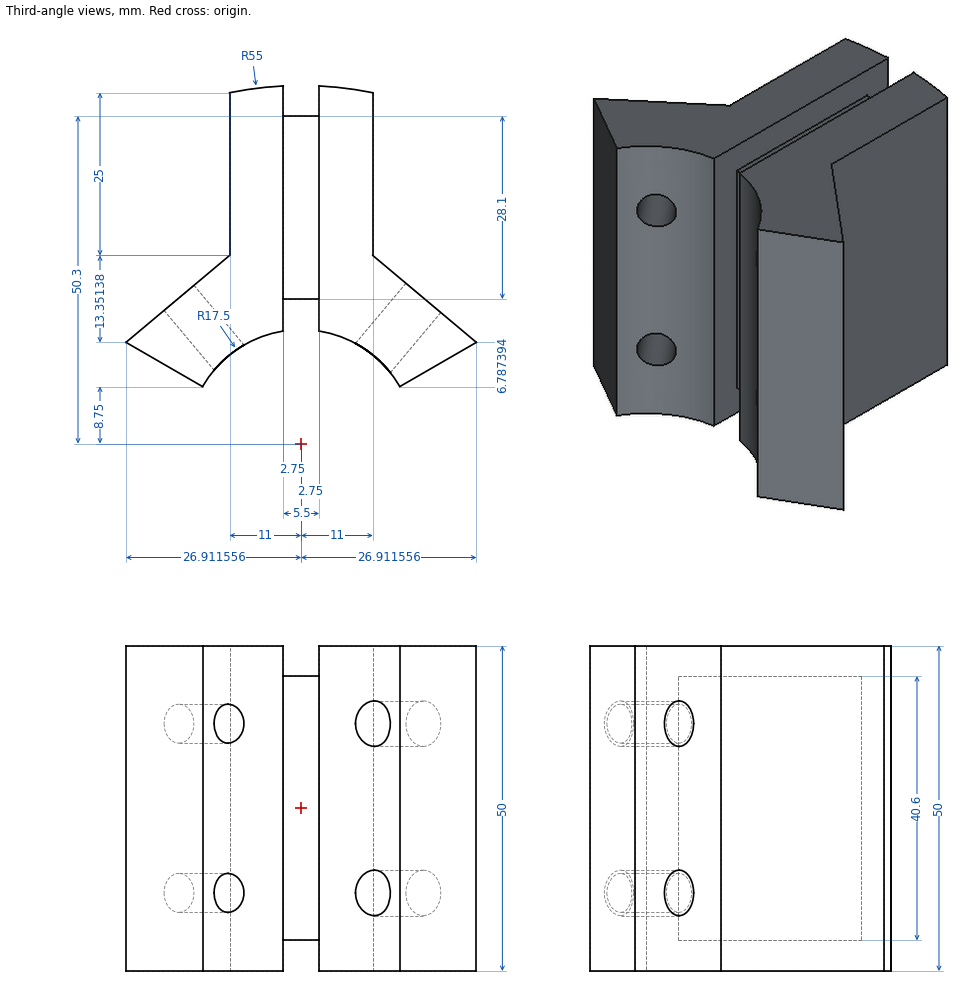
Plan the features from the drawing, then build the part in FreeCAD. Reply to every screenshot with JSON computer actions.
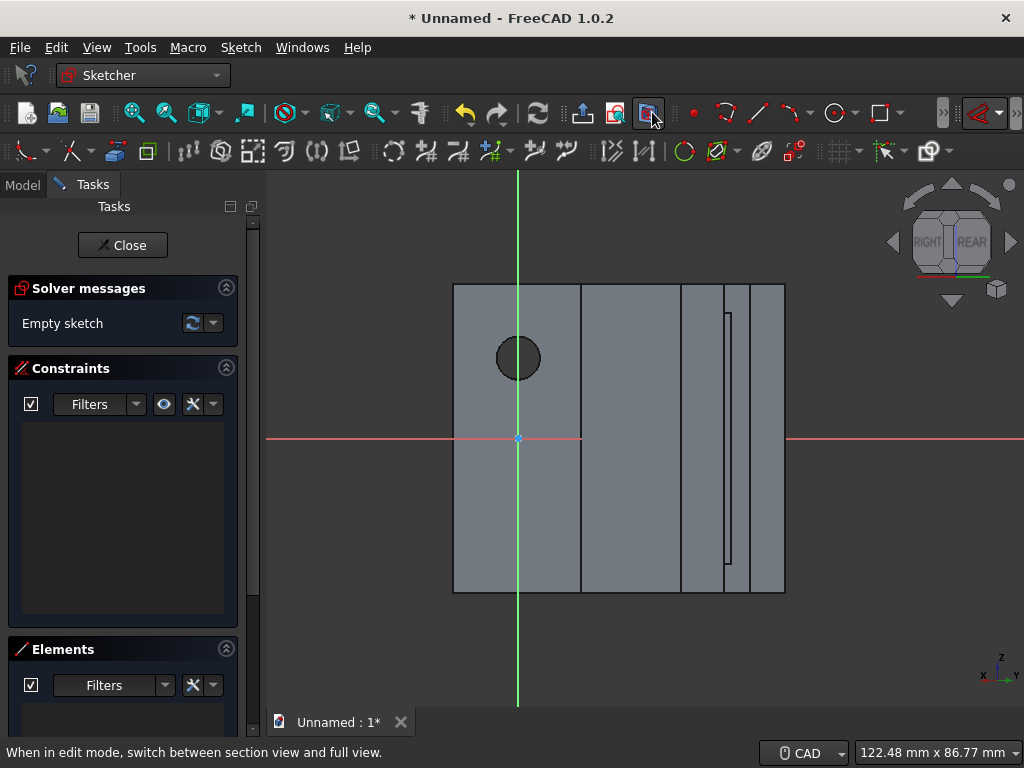
{"action": "scroll", "coordinate": [493, 512], "scroll_direction": "up", "scroll_amount": 6}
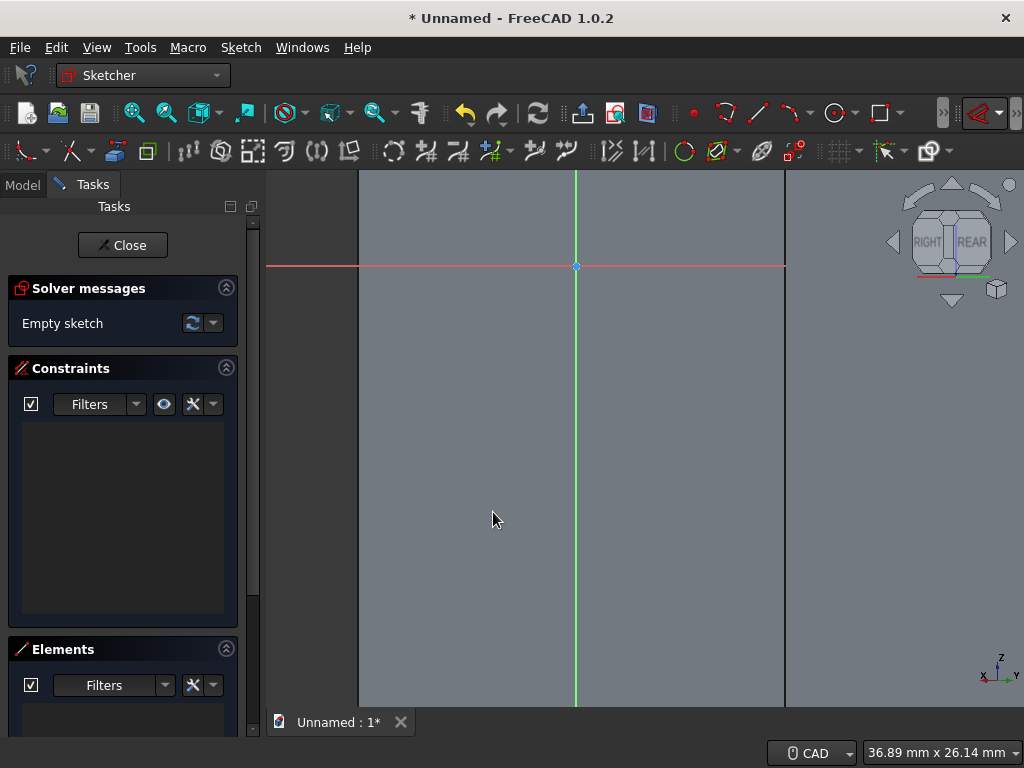
{"action": "key", "text": "g c"}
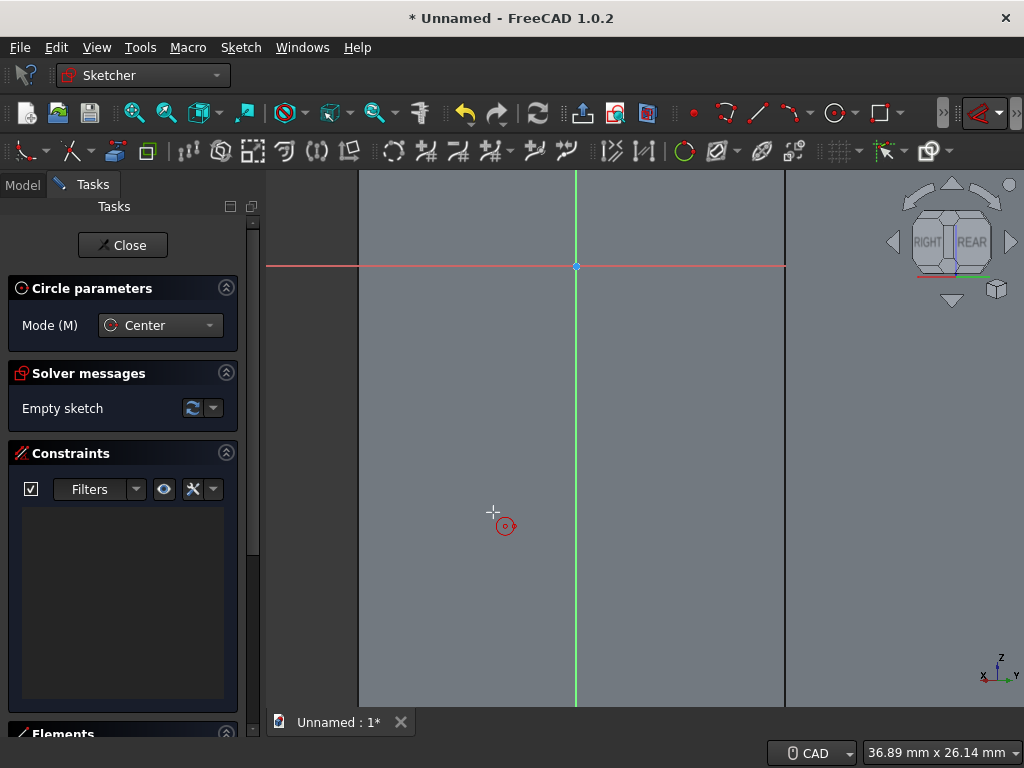
{"action": "left_click", "coordinate": [576, 534]}
{"action": "mouse_move", "coordinate": [627, 483]}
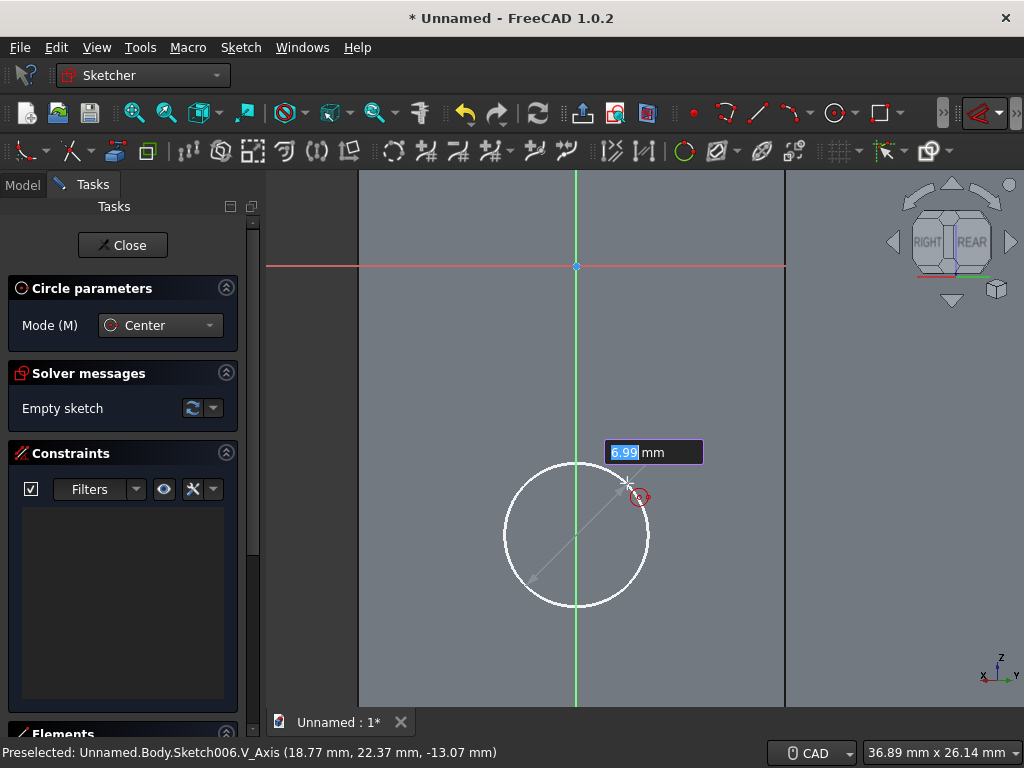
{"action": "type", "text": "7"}
{"action": "key", "text": "Return"}
{"action": "key", "text": "Escape"}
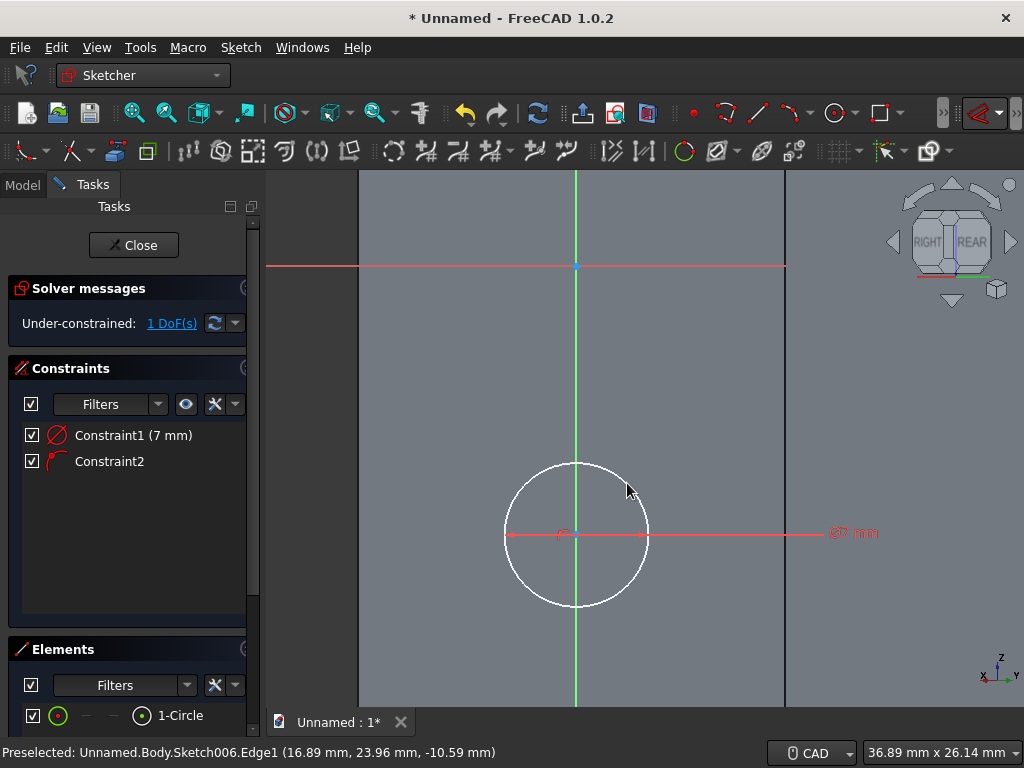
{"action": "left_click", "coordinate": [576, 535]}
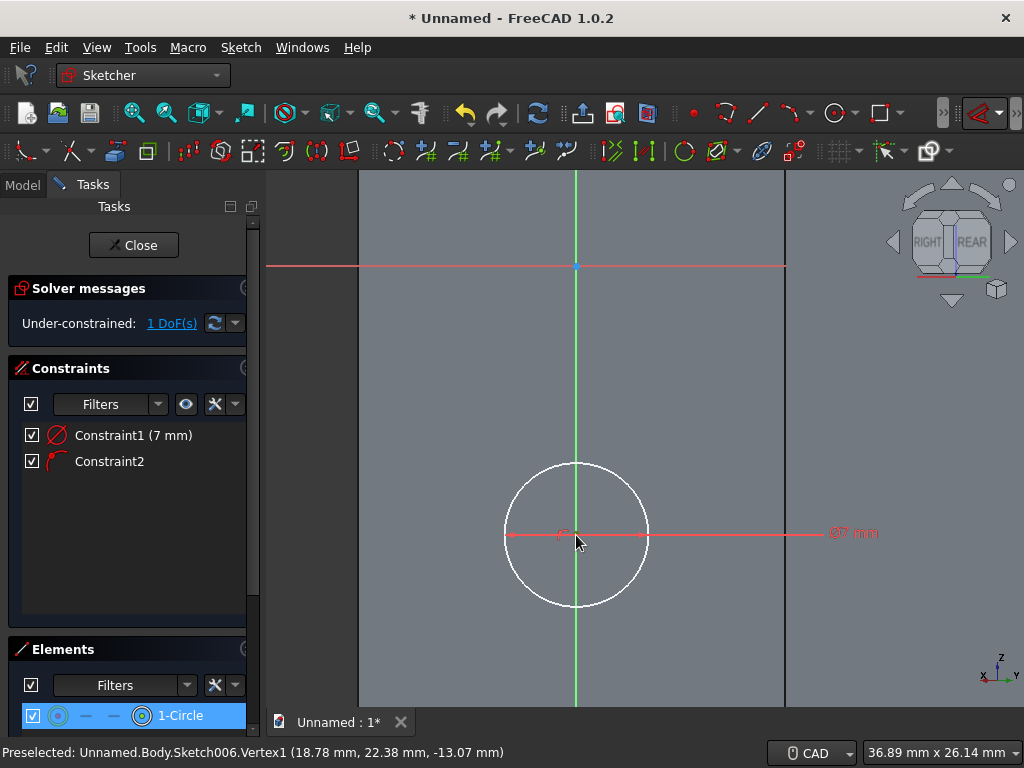
{"action": "key", "text": "i"}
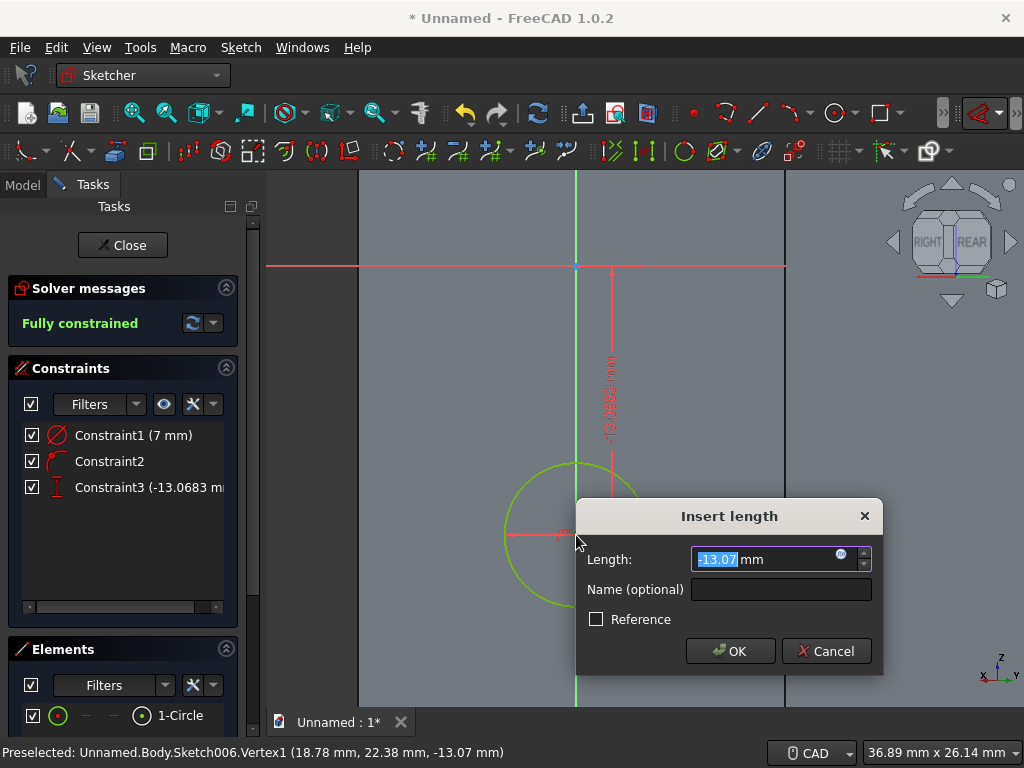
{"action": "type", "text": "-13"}
{"action": "key", "text": "Return"}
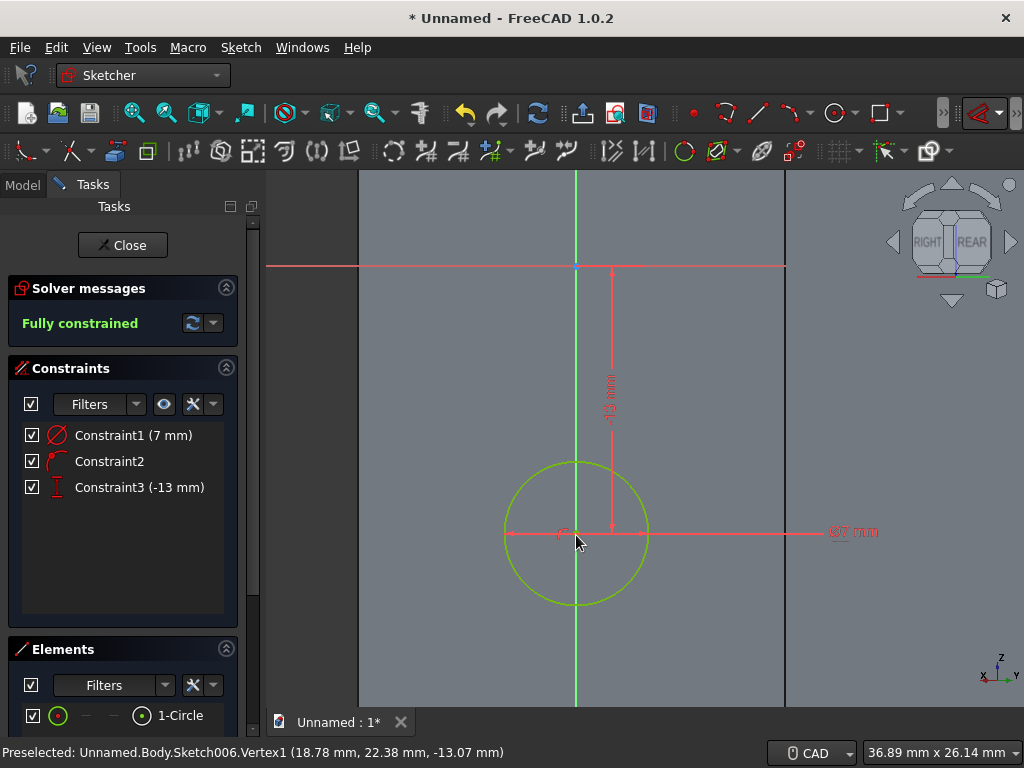
{"action": "left_click", "coordinate": [123, 245]}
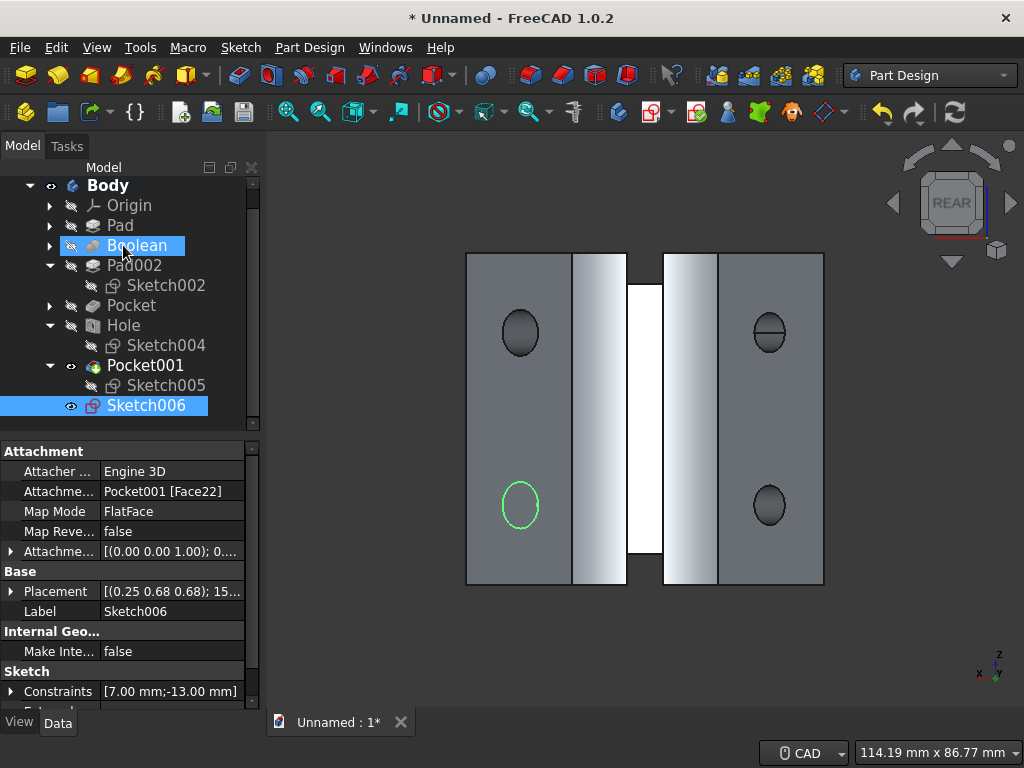
{"action": "left_click", "coordinate": [272, 76]}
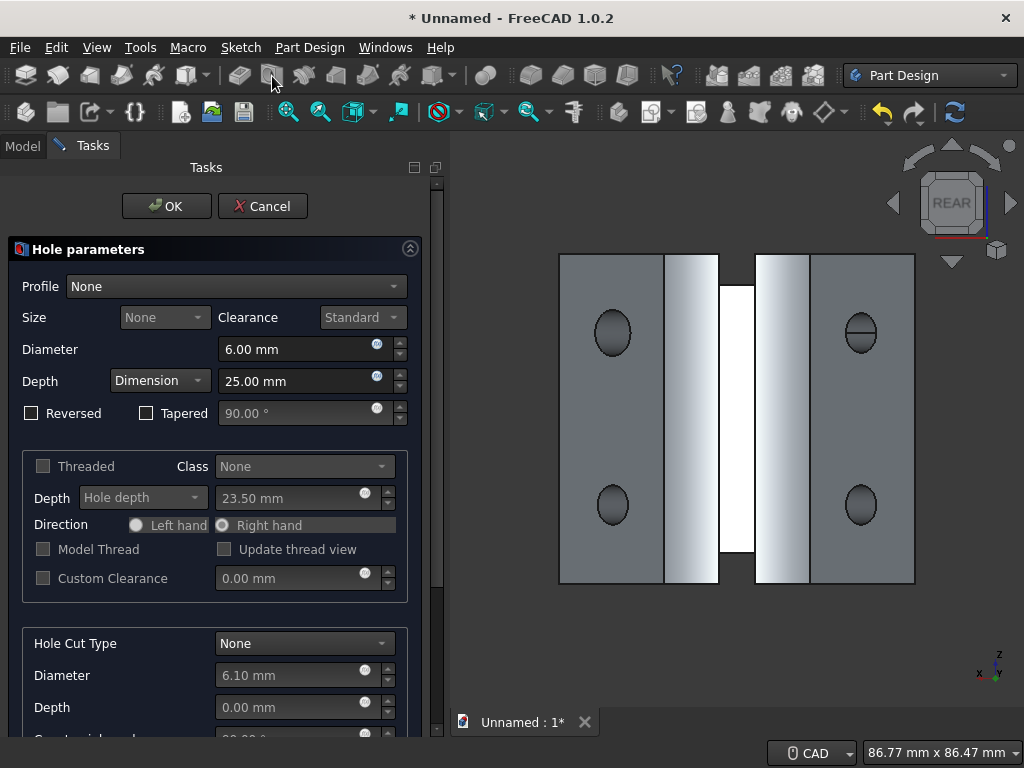
{"action": "triple_click", "coordinate": [305, 349]}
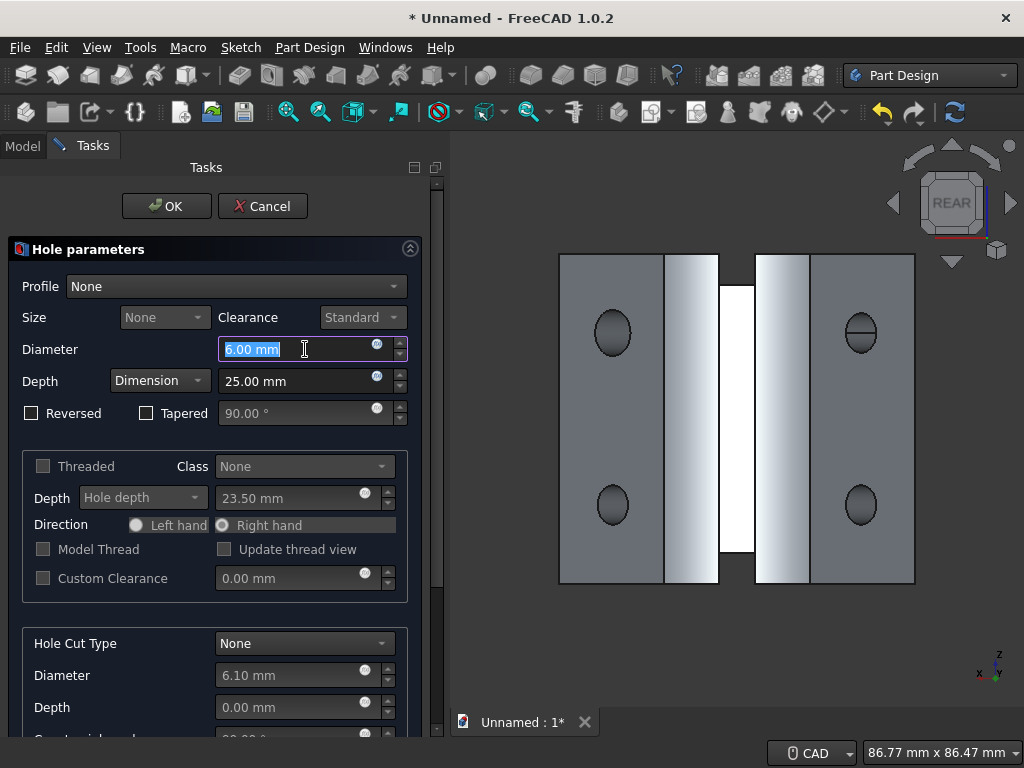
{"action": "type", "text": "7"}
{"action": "key", "text": "Tab"}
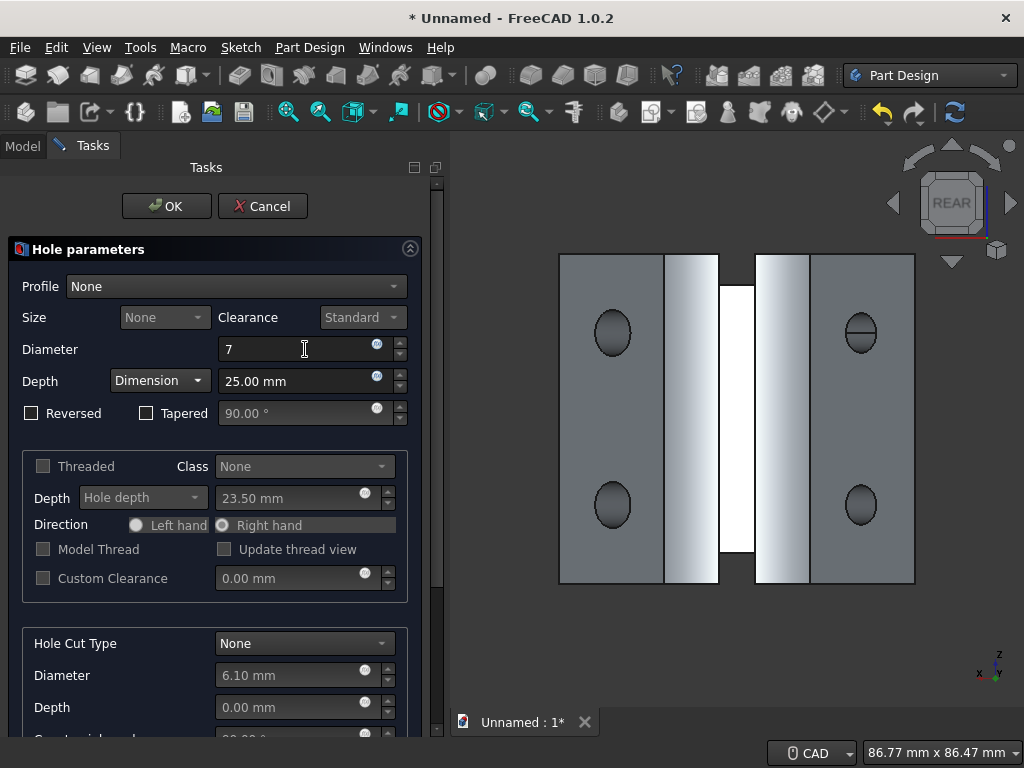
{"action": "left_click", "coordinate": [161, 380]}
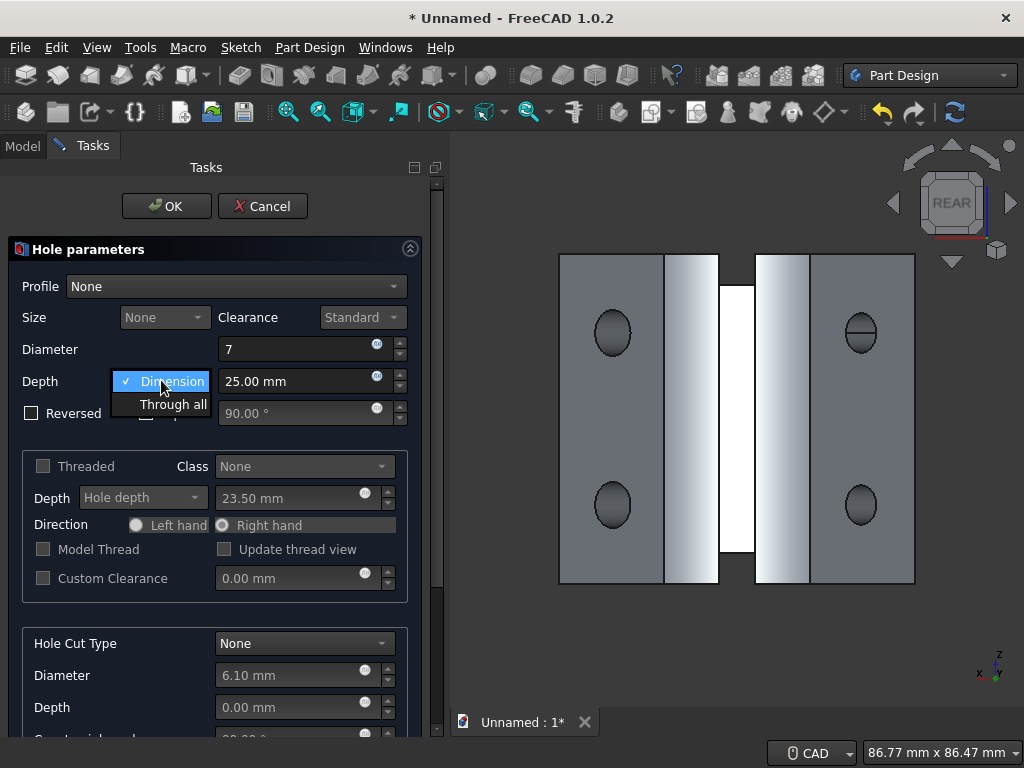
{"action": "left_click", "coordinate": [160, 404]}